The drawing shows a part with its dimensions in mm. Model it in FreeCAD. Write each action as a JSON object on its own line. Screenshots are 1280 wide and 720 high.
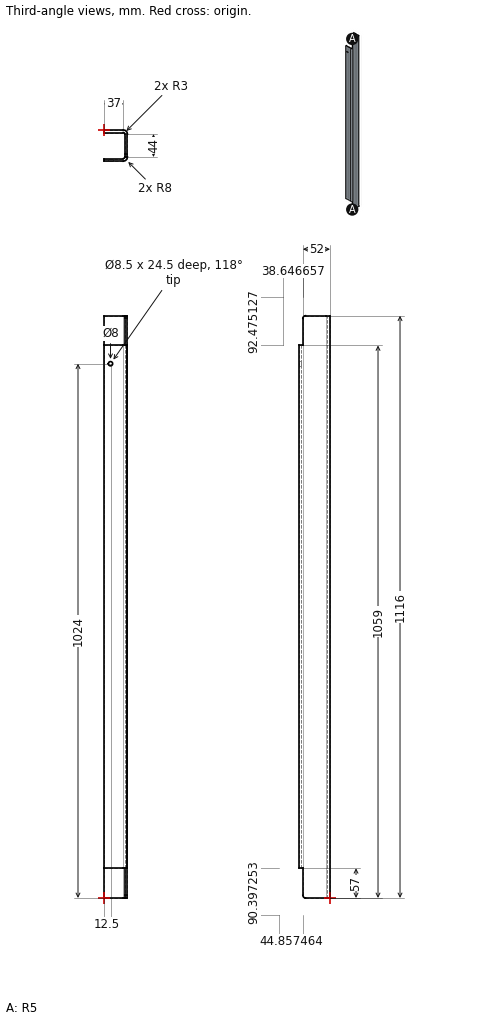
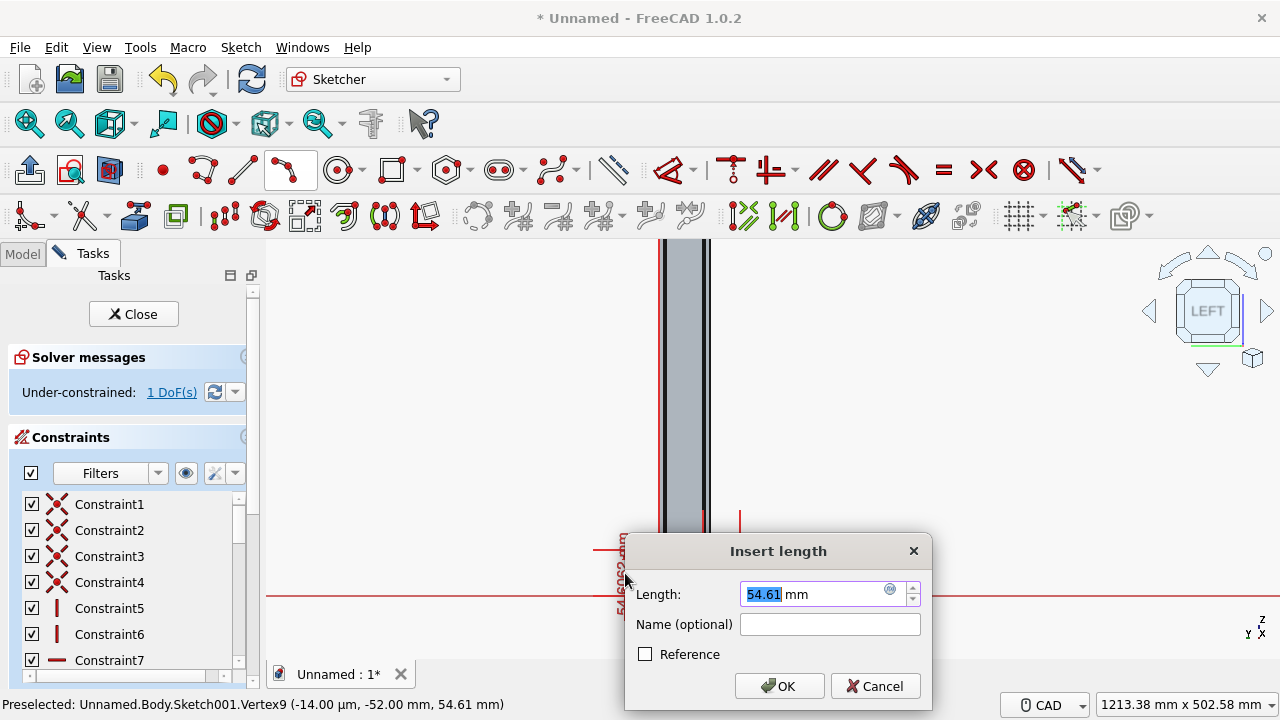
{"action": "type", "text": "57"}
{"action": "key", "text": "Return"}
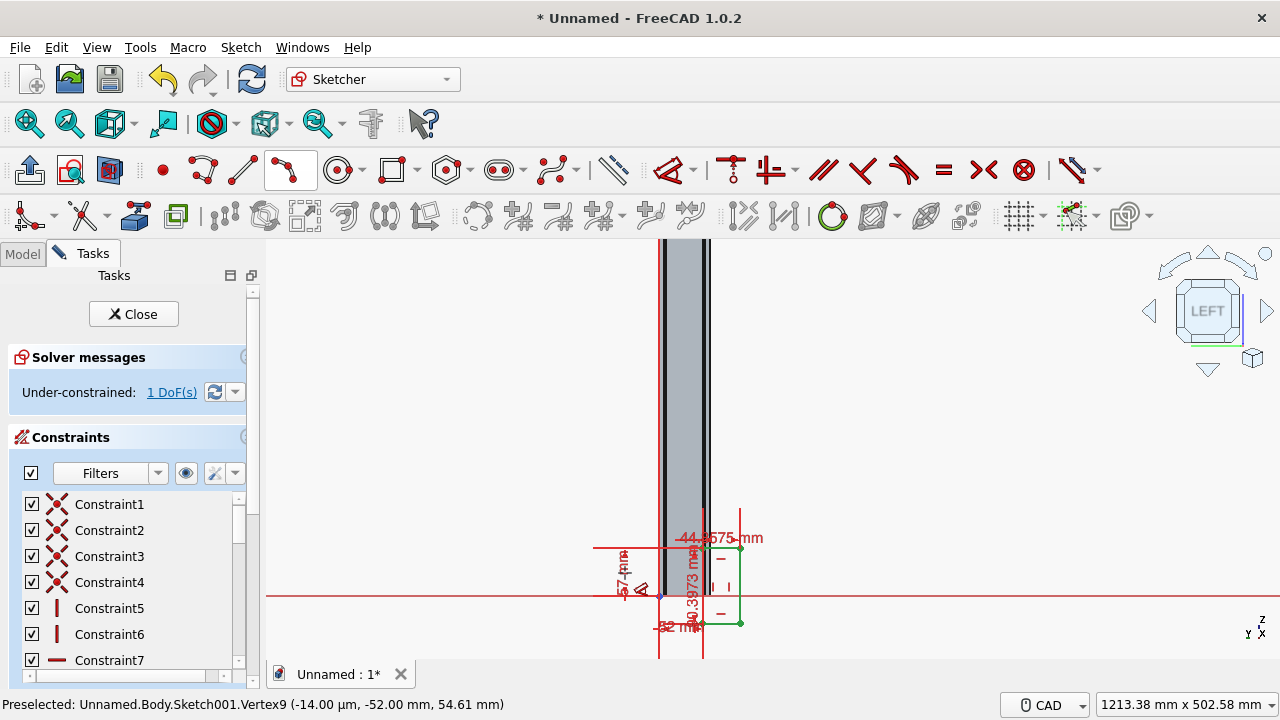
{"action": "scroll", "coordinate": [706, 554], "scroll_direction": "down", "scroll_amount": 7}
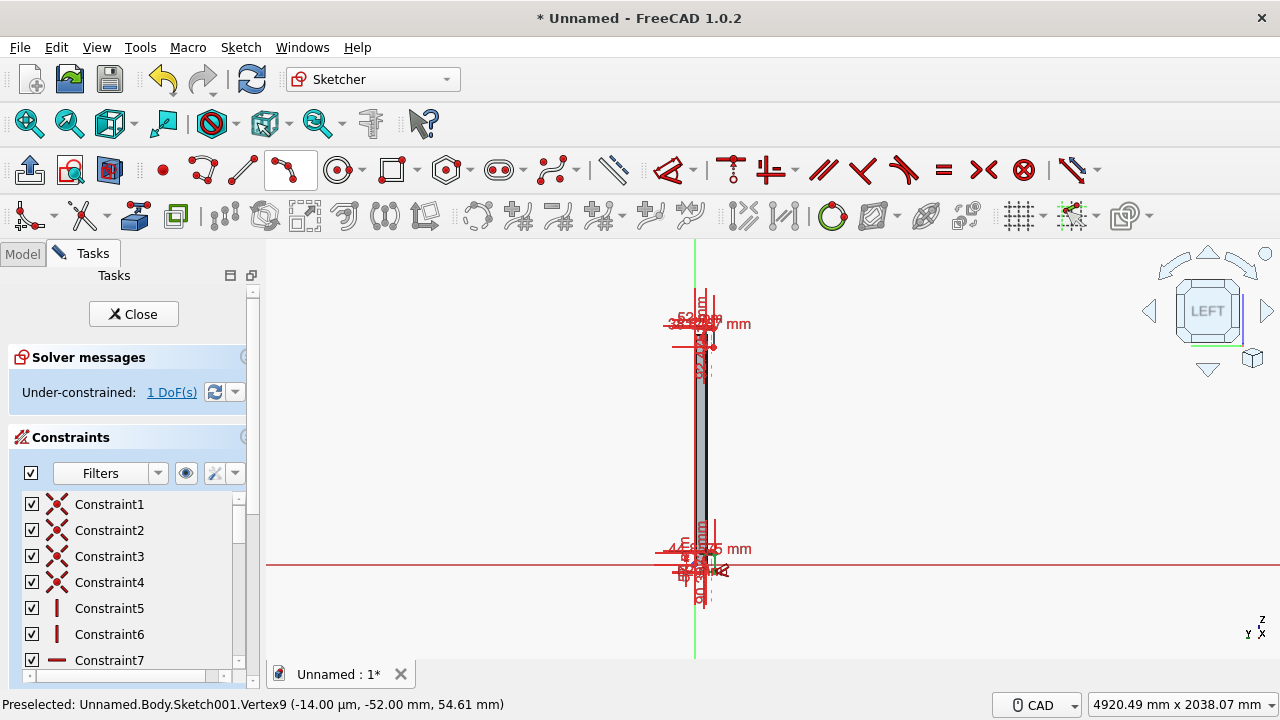
{"action": "scroll", "coordinate": [706, 347], "scroll_direction": "up", "scroll_amount": 3}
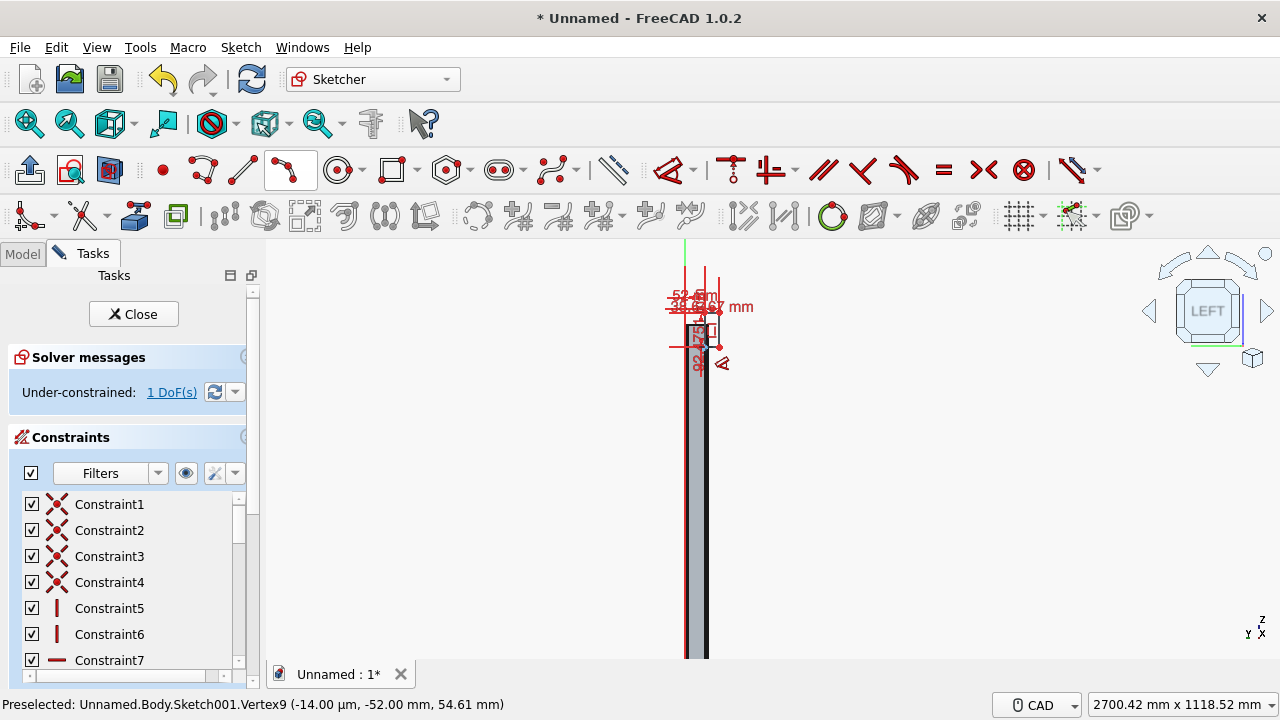
{"action": "left_click", "coordinate": [705, 347]}
{"action": "left_click", "coordinate": [651, 489]}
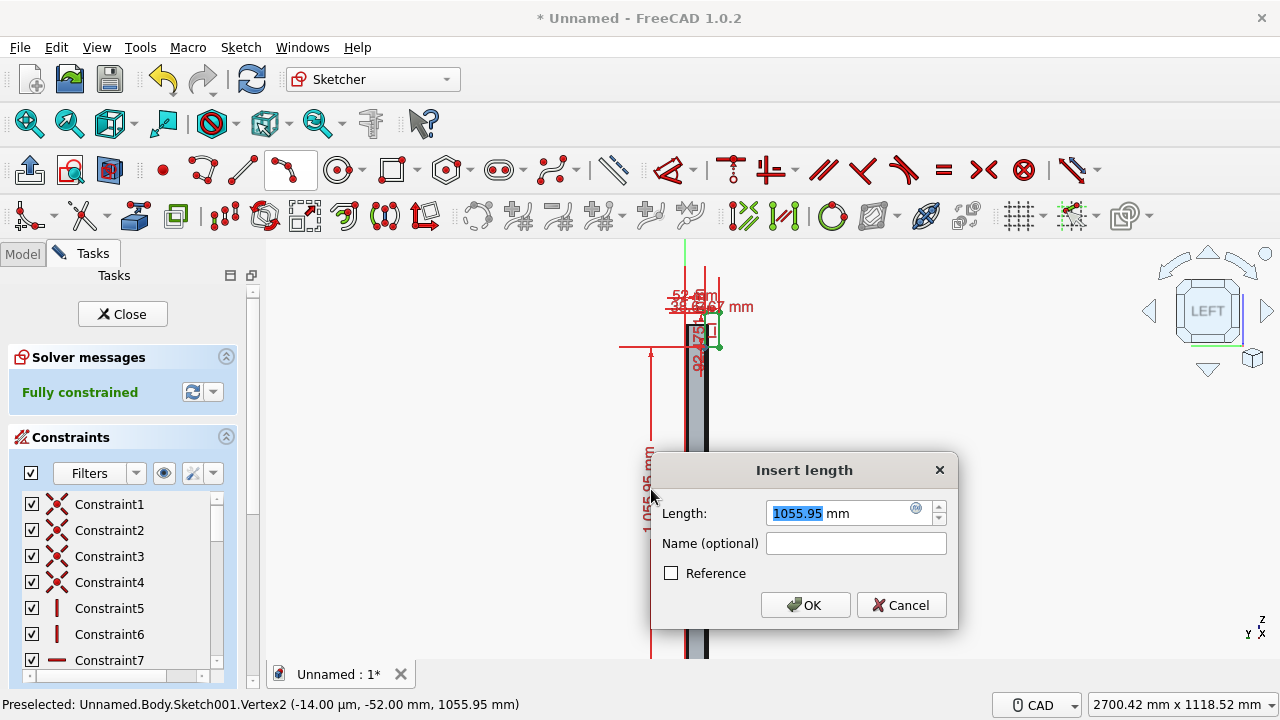
{"action": "type", "text": "1059"}
{"action": "key", "text": "Return"}
{"action": "key", "text": "Escape"}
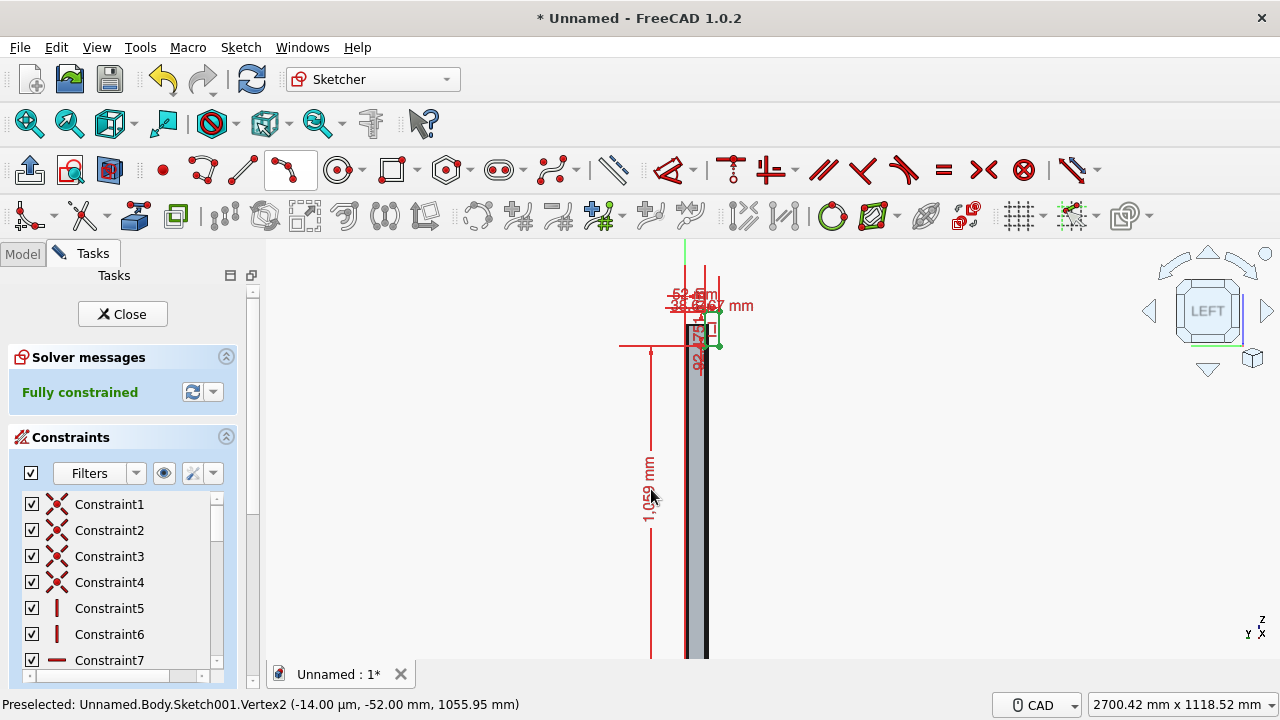
{"action": "left_click", "coordinate": [123, 314]}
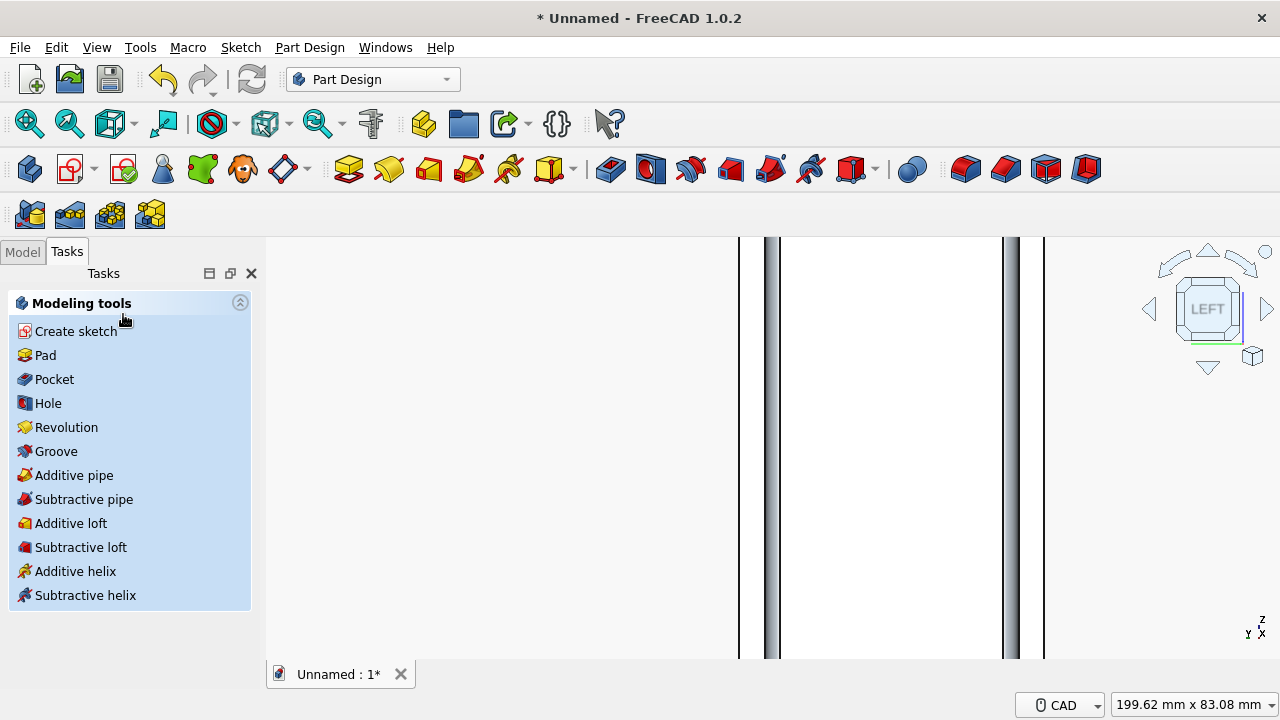
{"action": "left_click", "coordinate": [612, 170]}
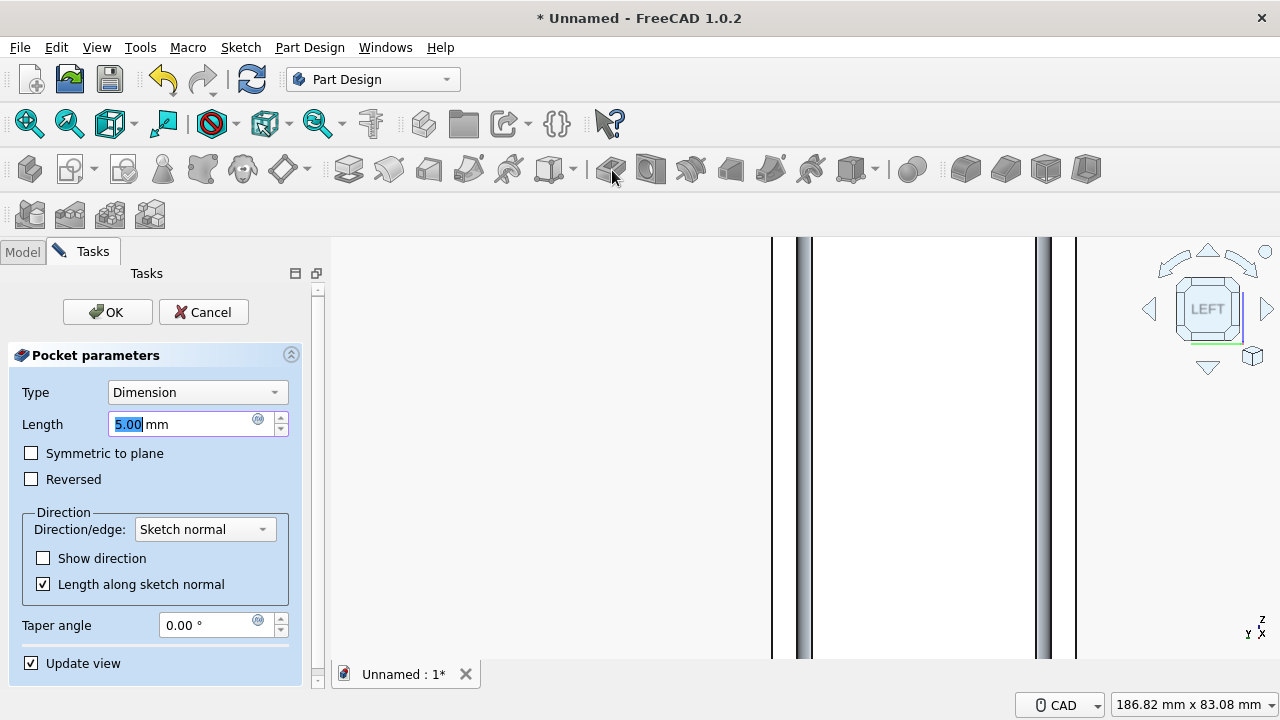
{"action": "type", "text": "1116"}
{"action": "key", "text": "Tab"}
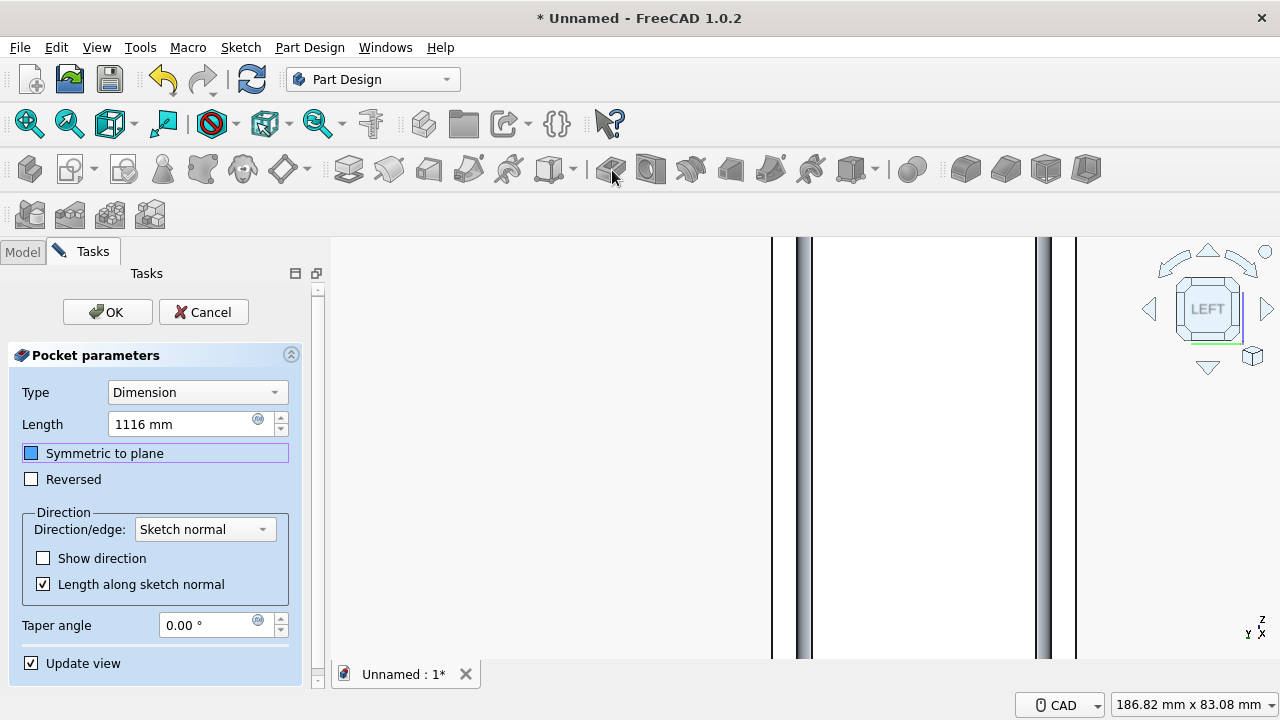
{"action": "left_click", "coordinate": [108, 312]}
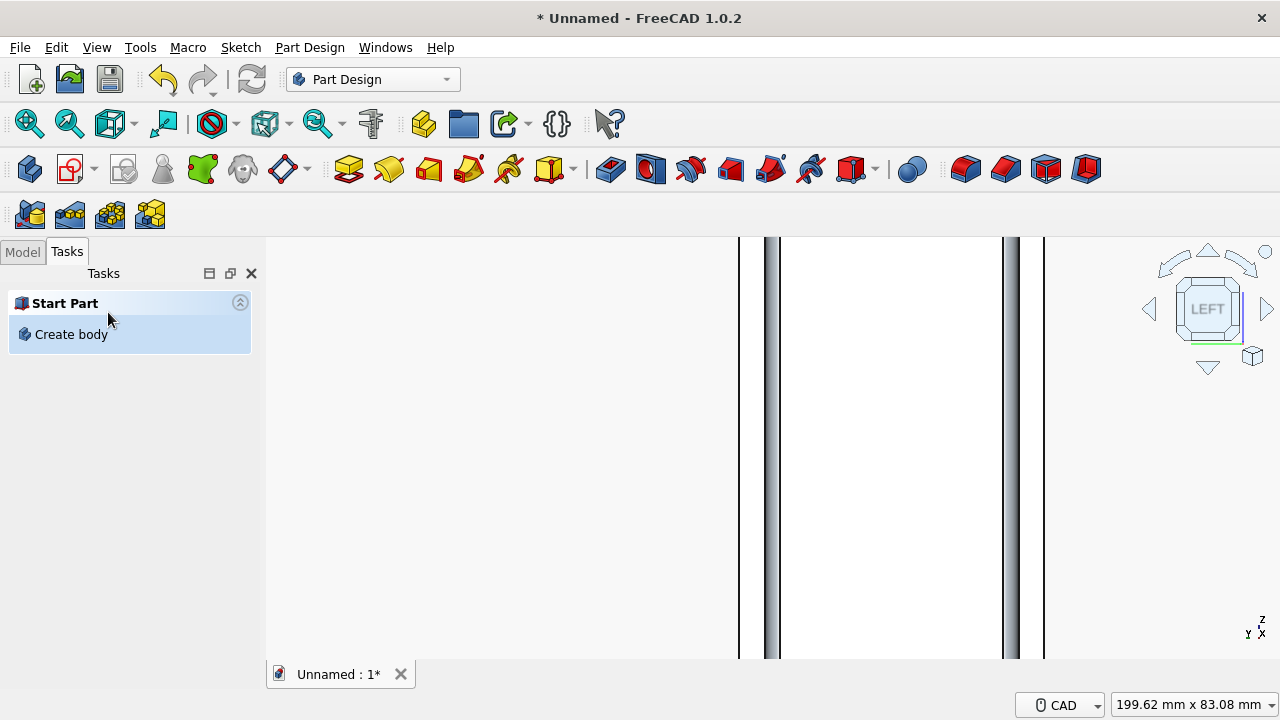
{"action": "left_click", "coordinate": [30, 124]}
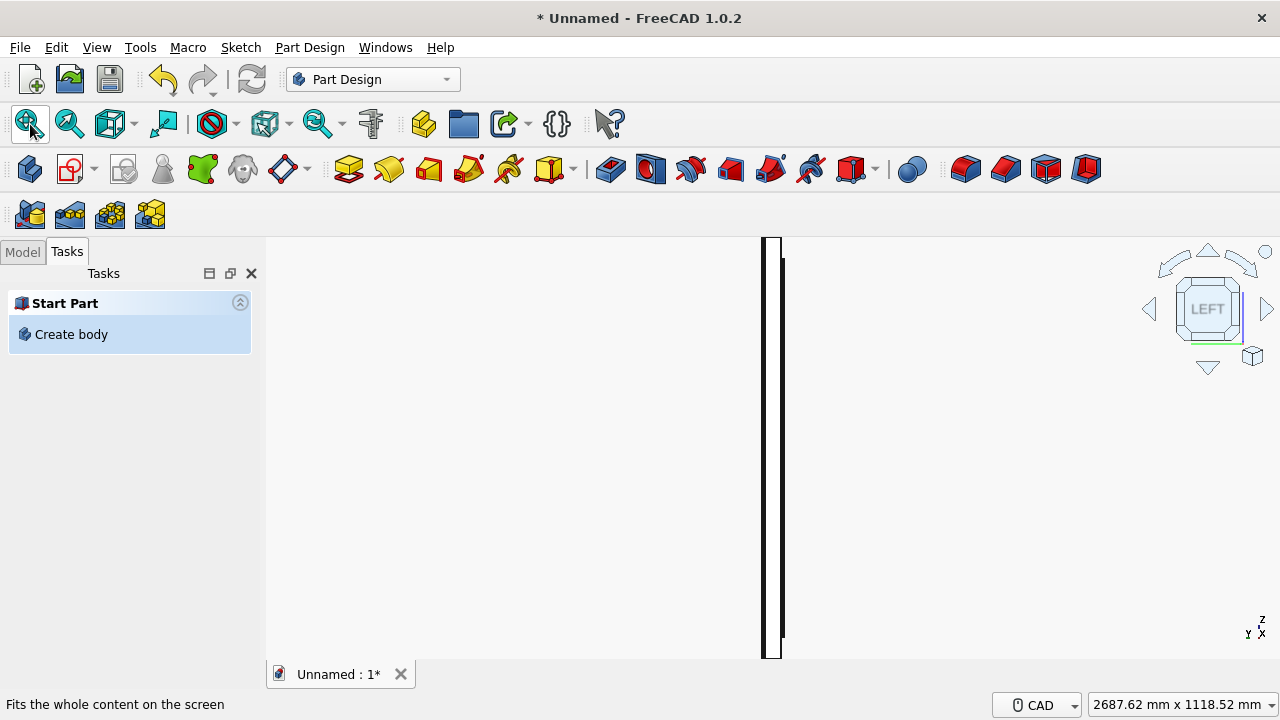
{"action": "left_click", "coordinate": [23, 251]}